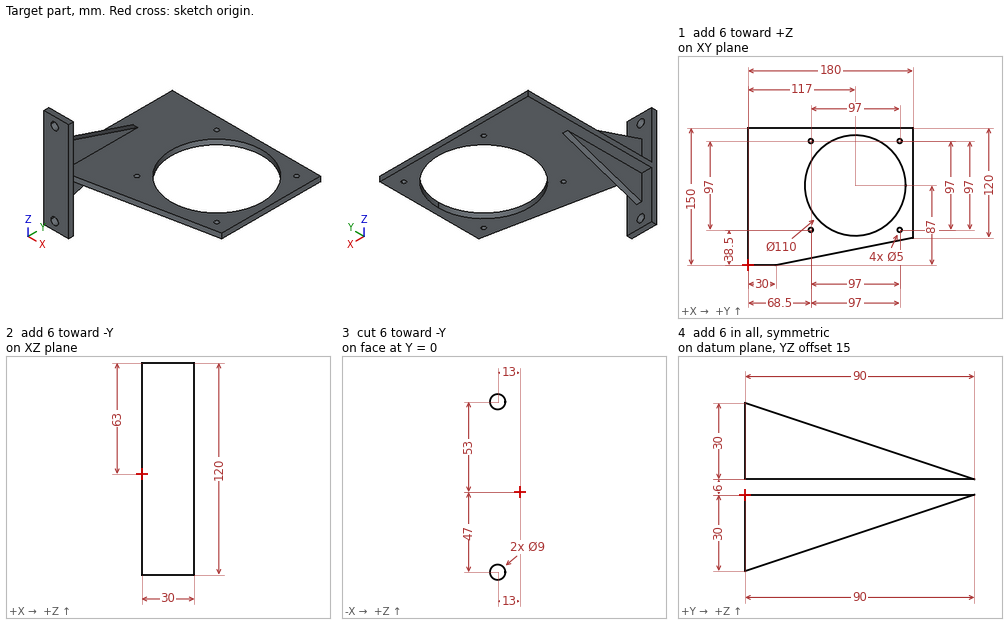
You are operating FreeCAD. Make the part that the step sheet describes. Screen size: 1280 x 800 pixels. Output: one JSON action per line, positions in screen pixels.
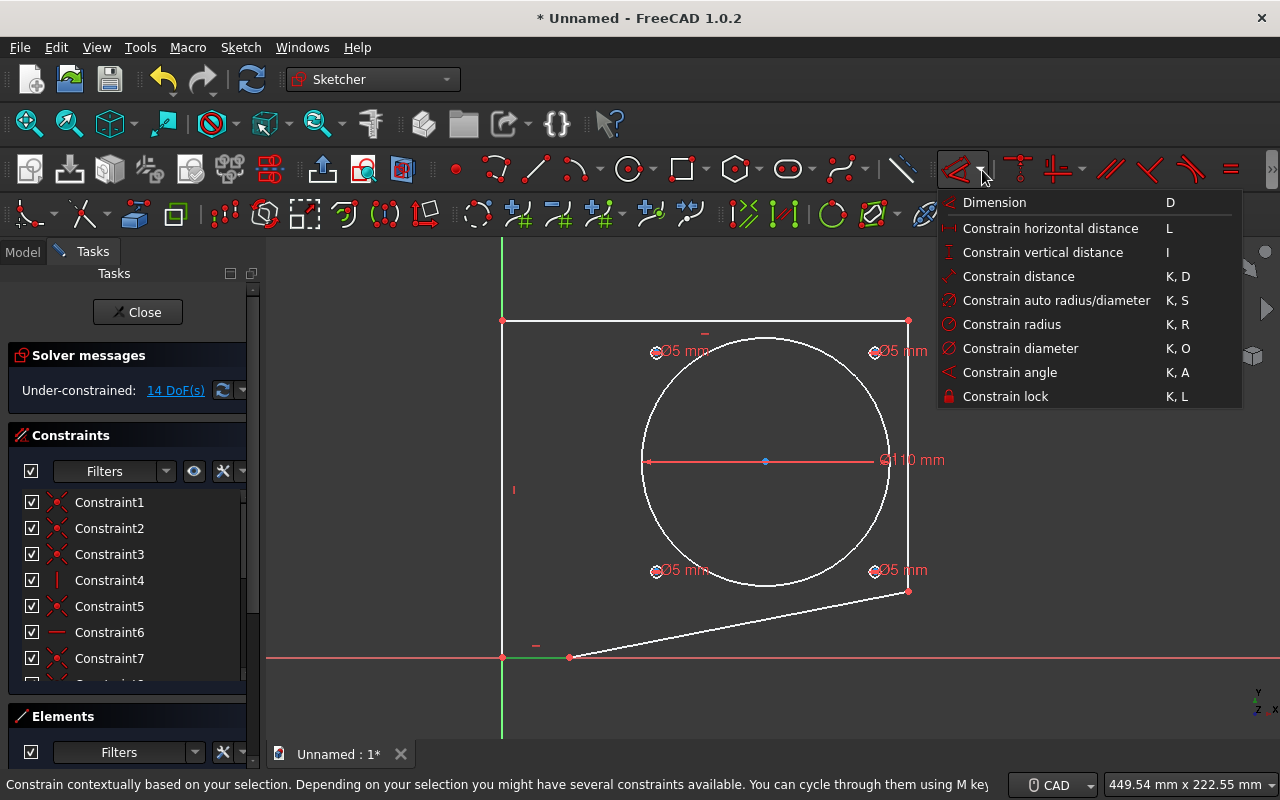
{"action": "left_click", "coordinate": [1090, 228]}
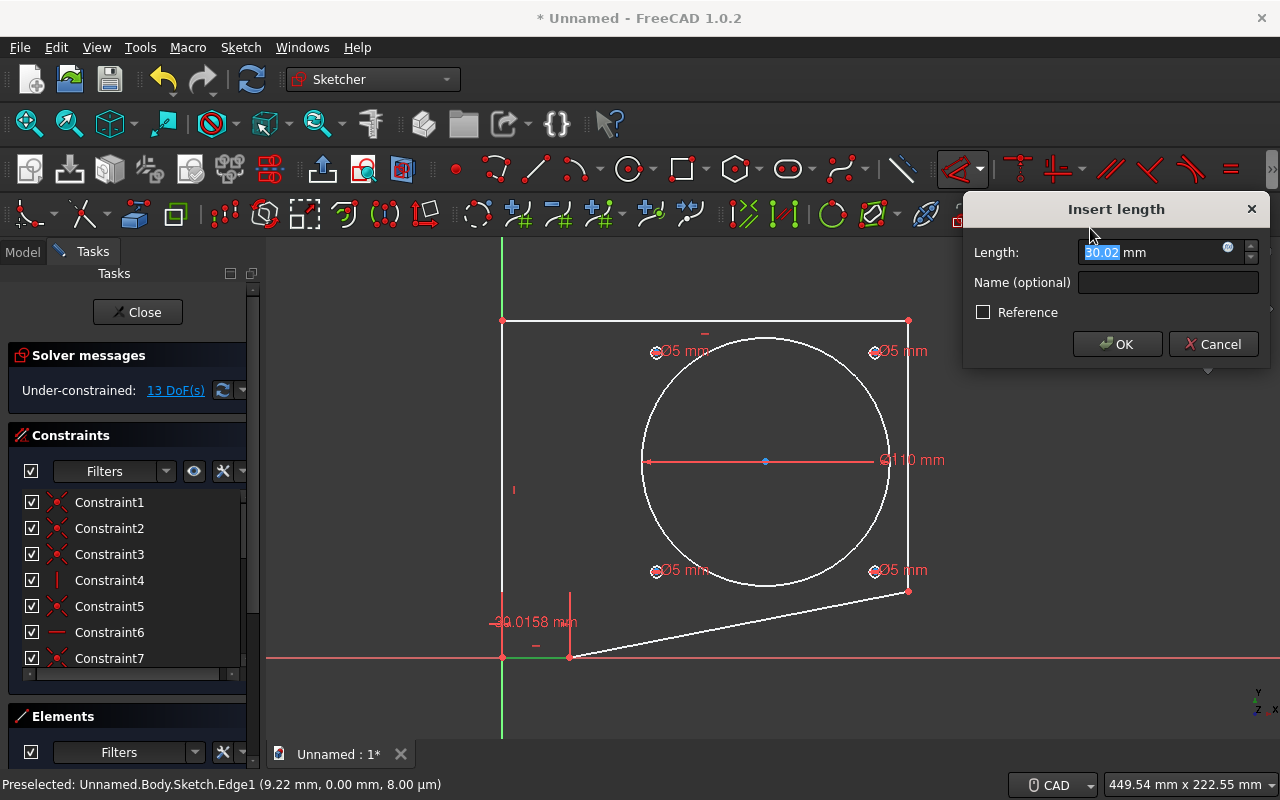
{"action": "type", "text": "30"}
{"action": "key", "text": "Return"}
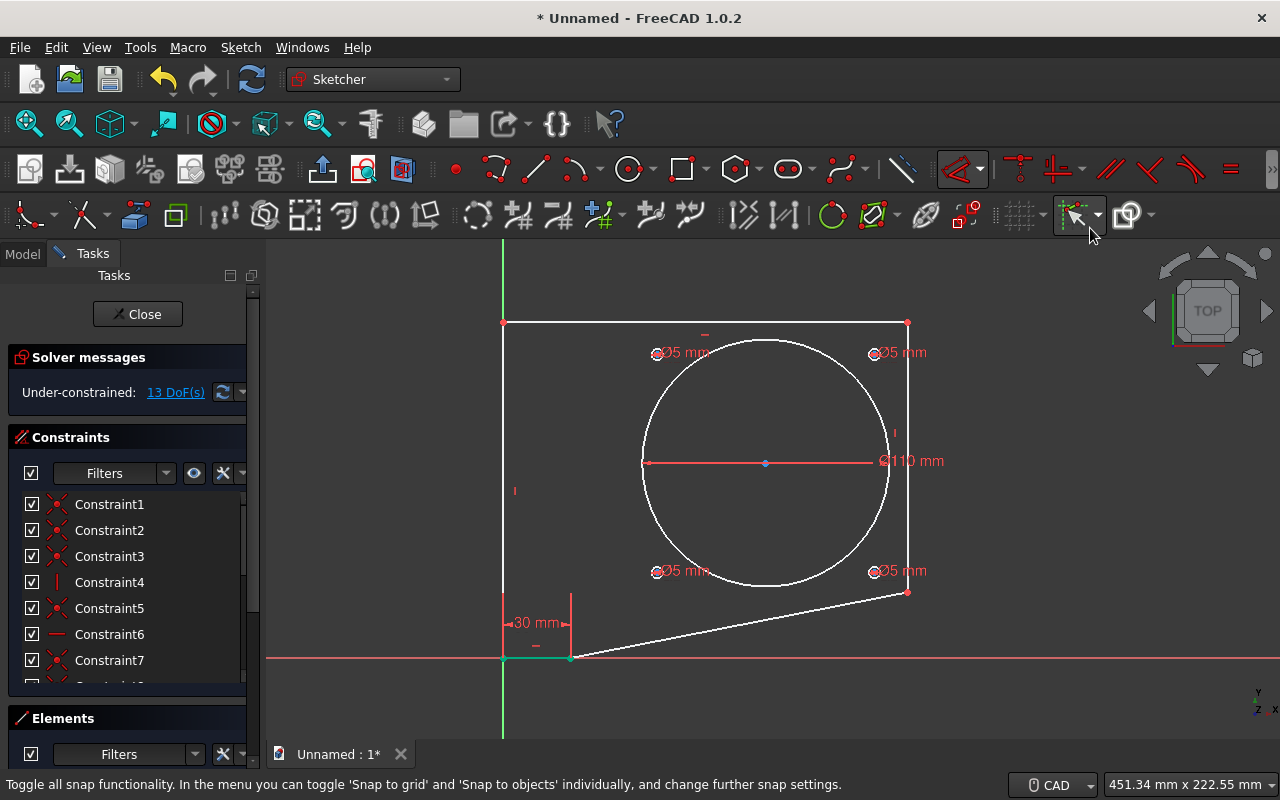
{"action": "left_click", "coordinate": [766, 463]}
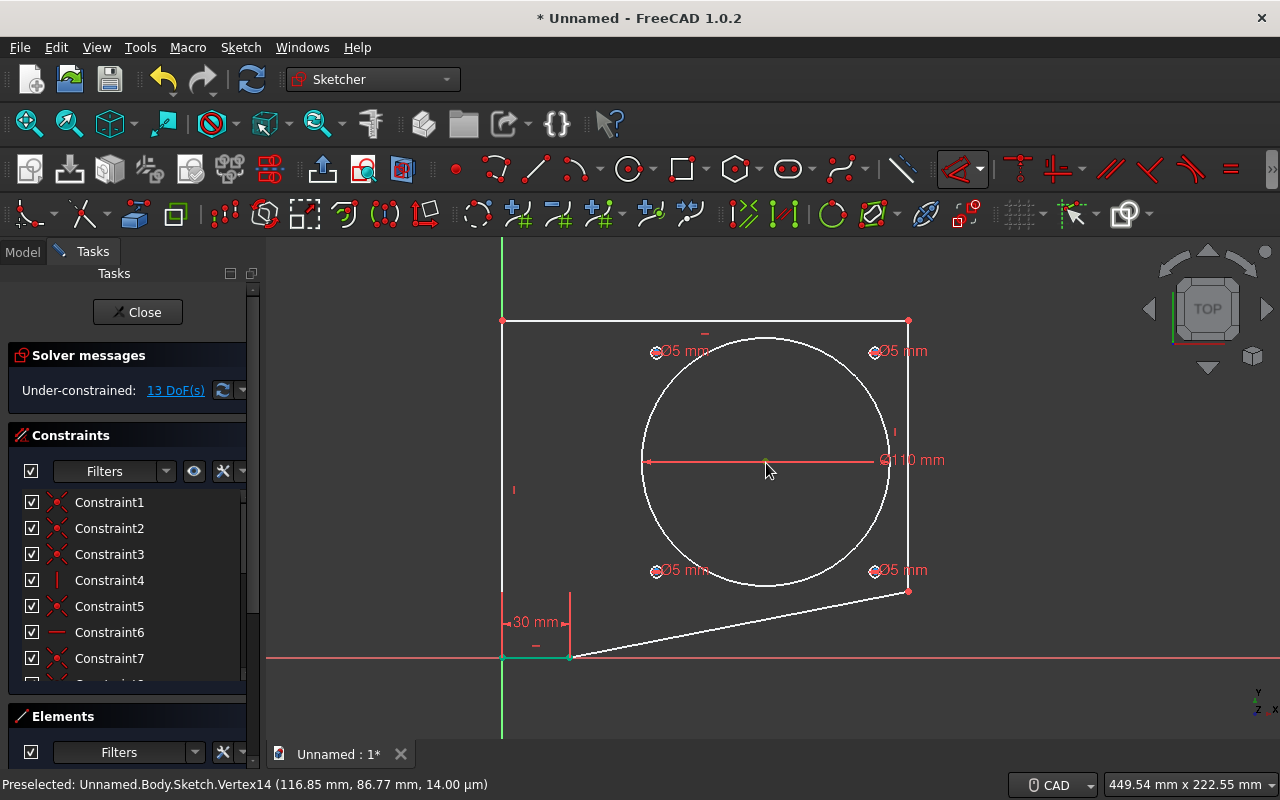
{"action": "key", "text": "i"}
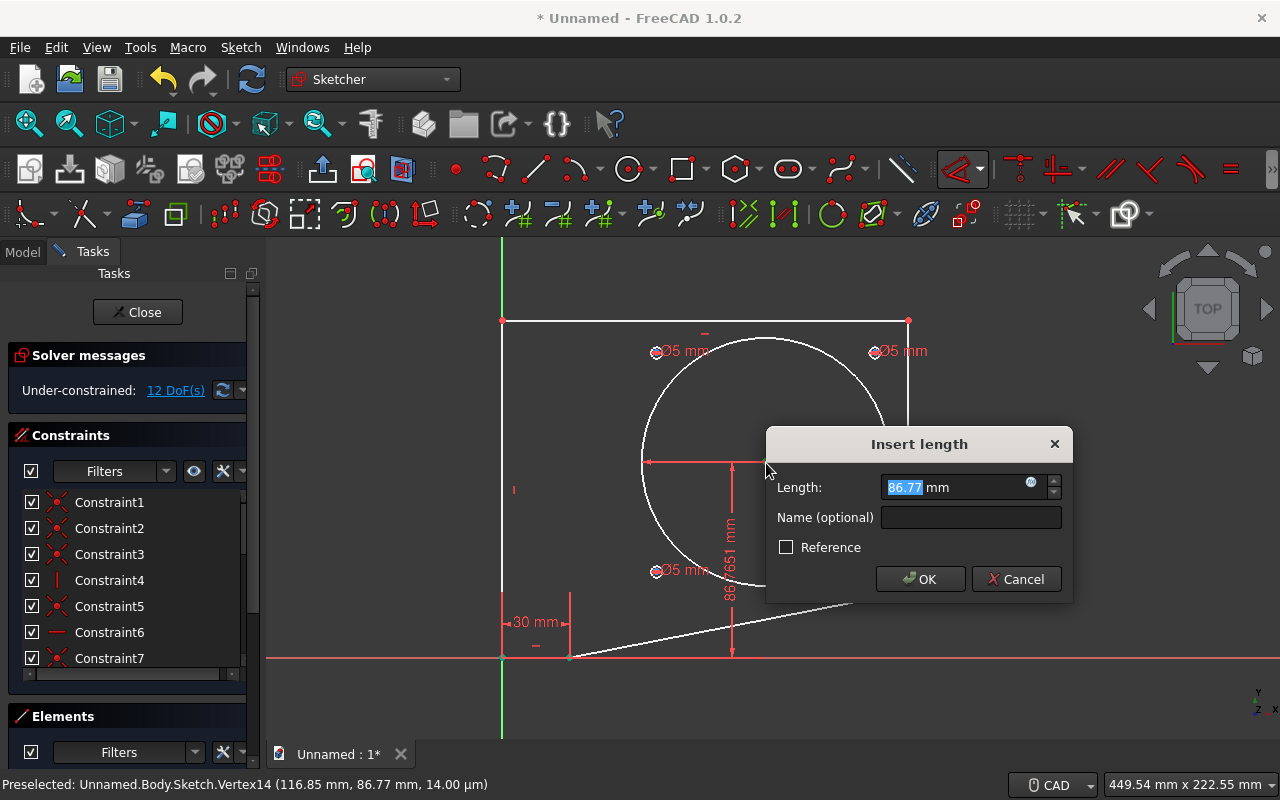
{"action": "type", "text": "87"}
{"action": "key", "text": "Return"}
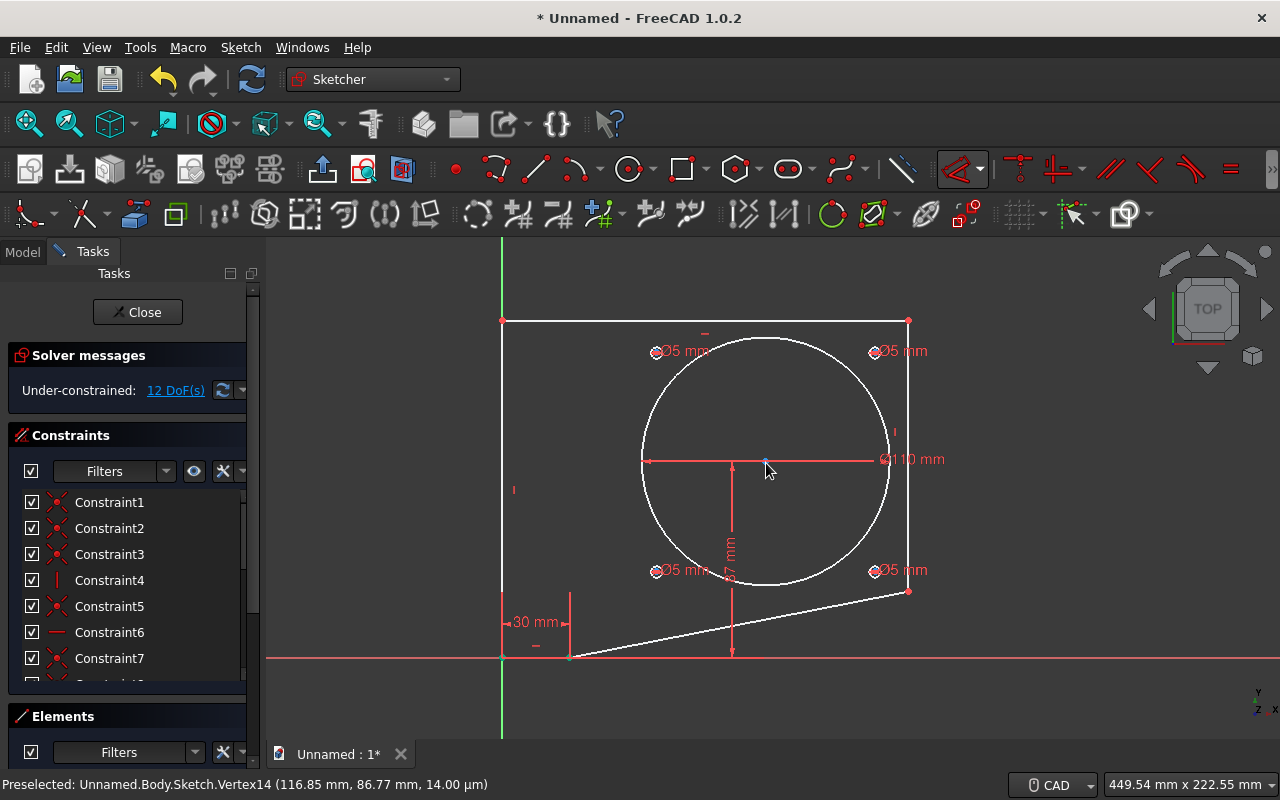
{"action": "left_click", "coordinate": [908, 510]}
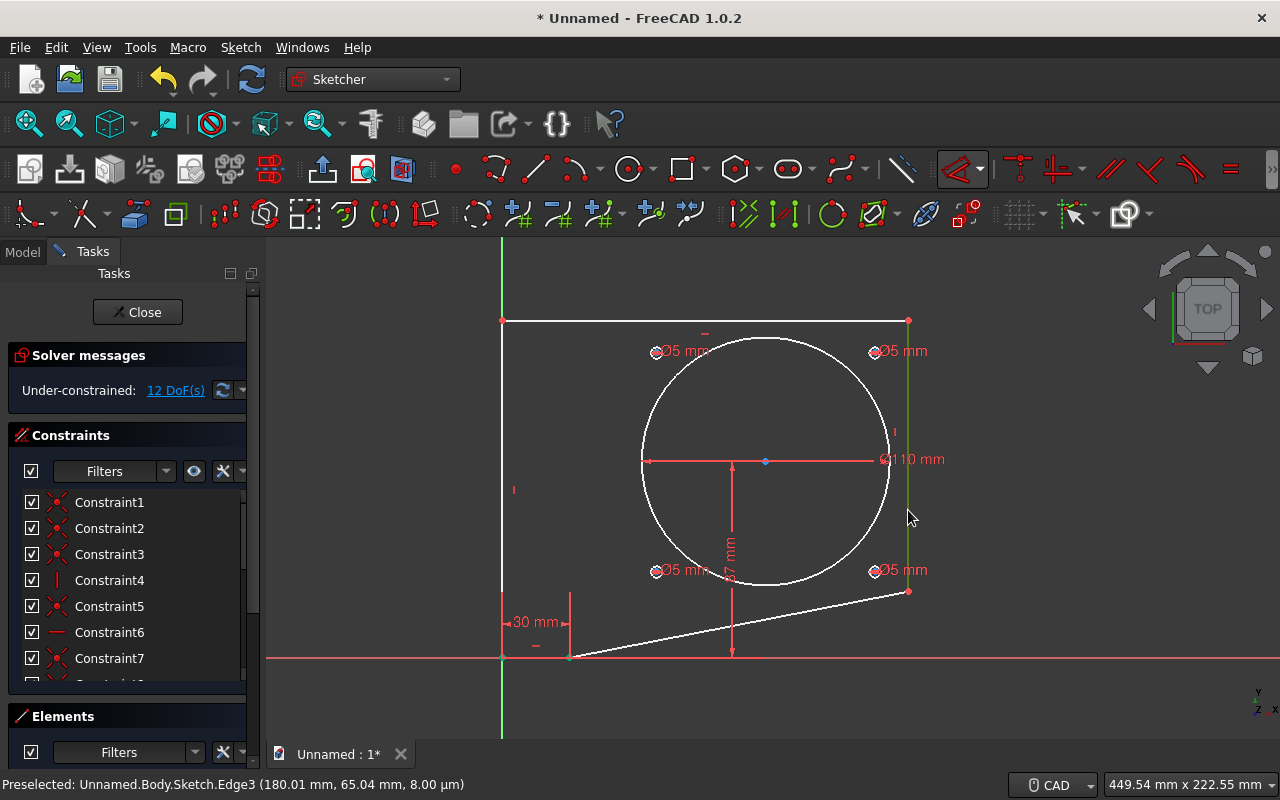
{"action": "key", "text": "i"}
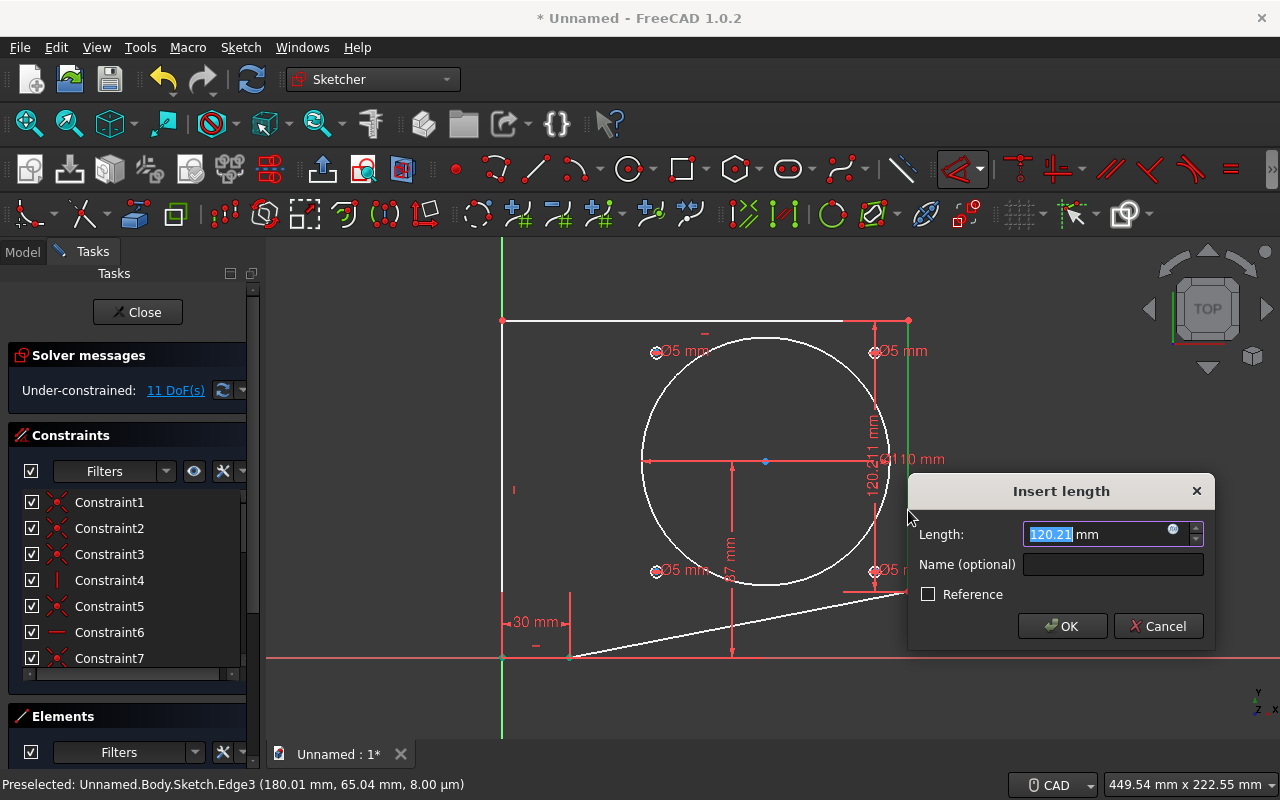
{"action": "type", "text": "120"}
{"action": "key", "text": "Return"}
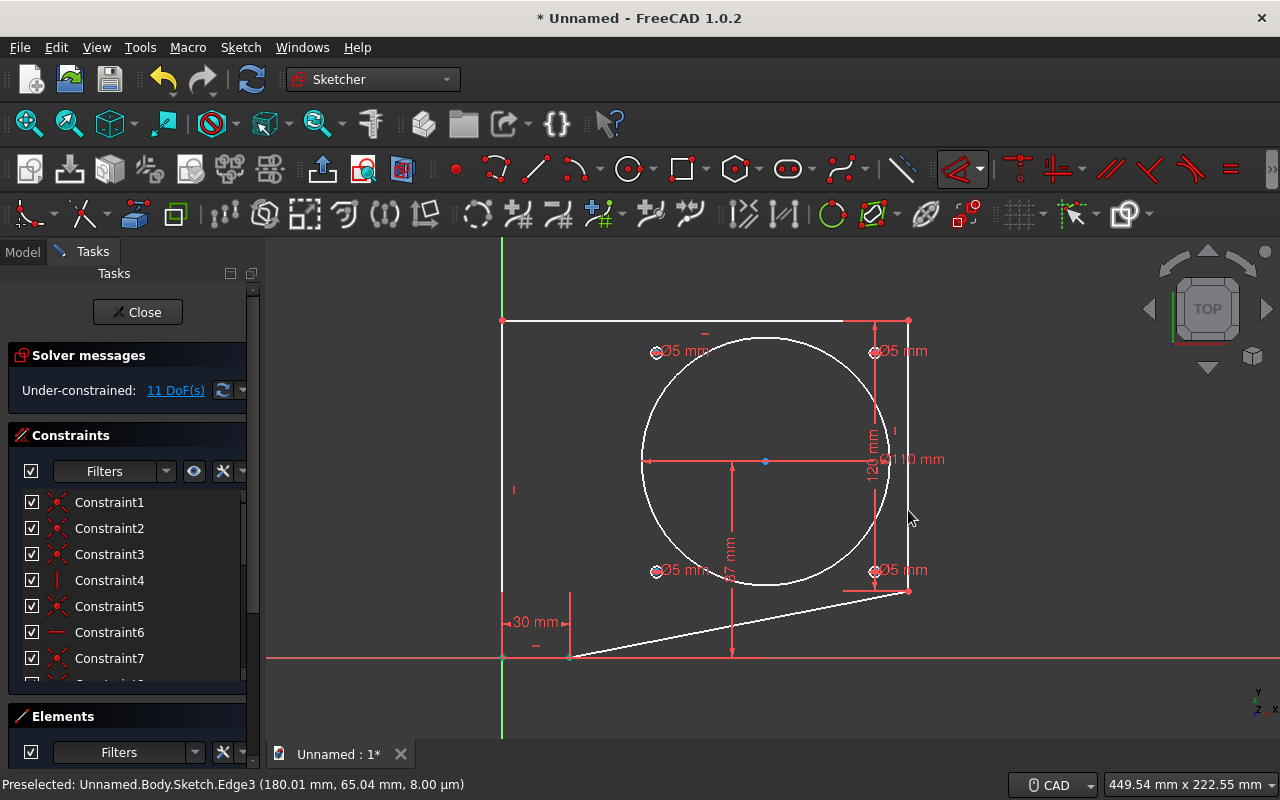
{"action": "left_click", "coordinate": [786, 321]}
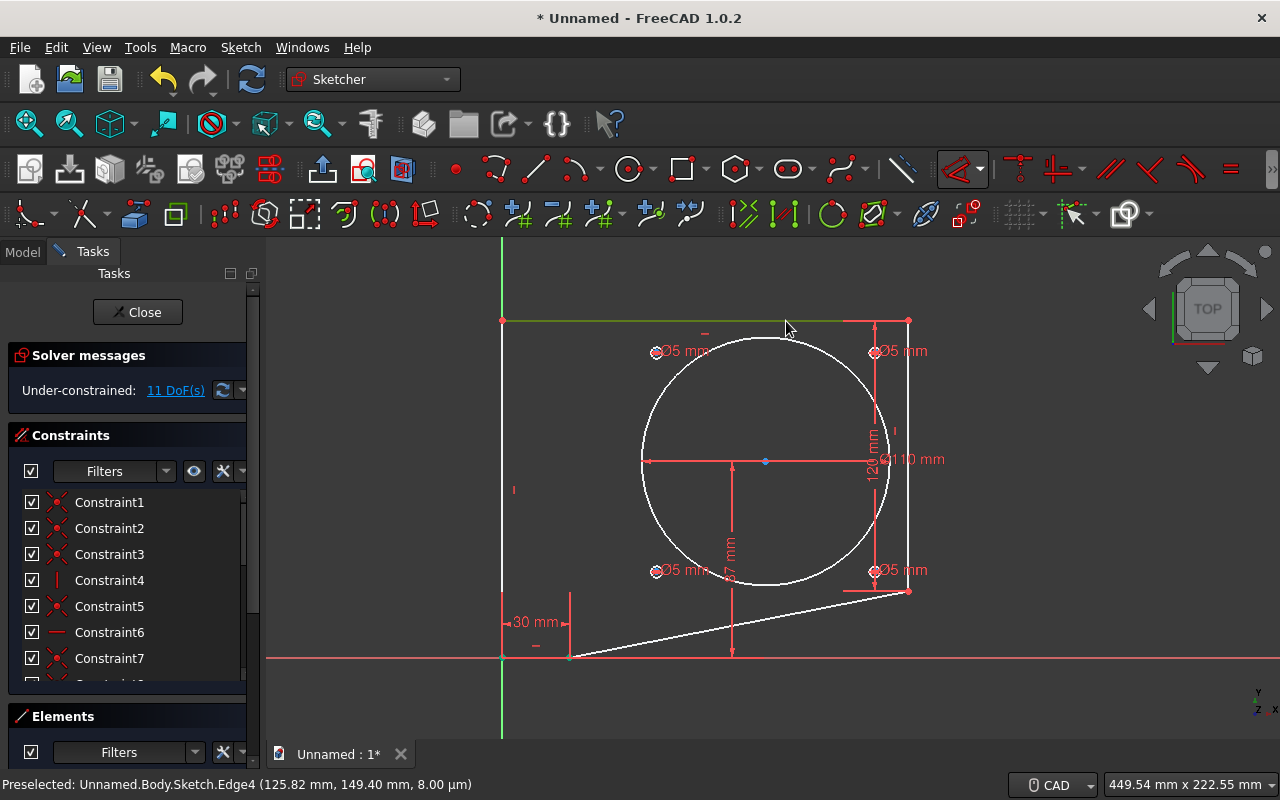
{"action": "key", "text": "l"}